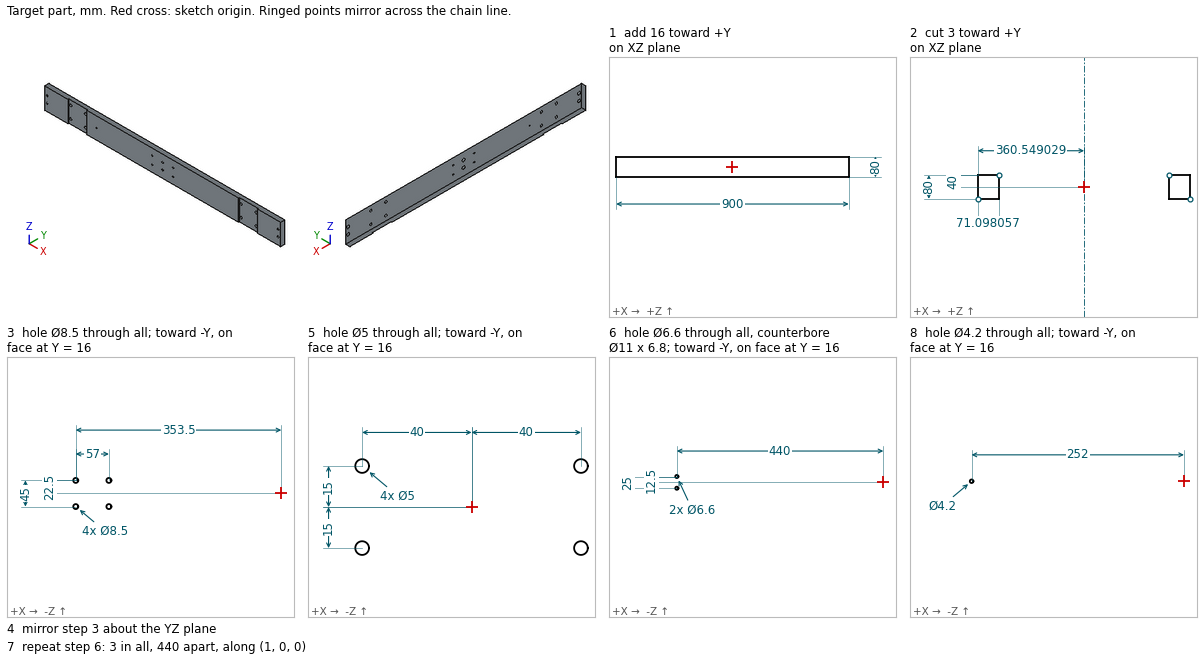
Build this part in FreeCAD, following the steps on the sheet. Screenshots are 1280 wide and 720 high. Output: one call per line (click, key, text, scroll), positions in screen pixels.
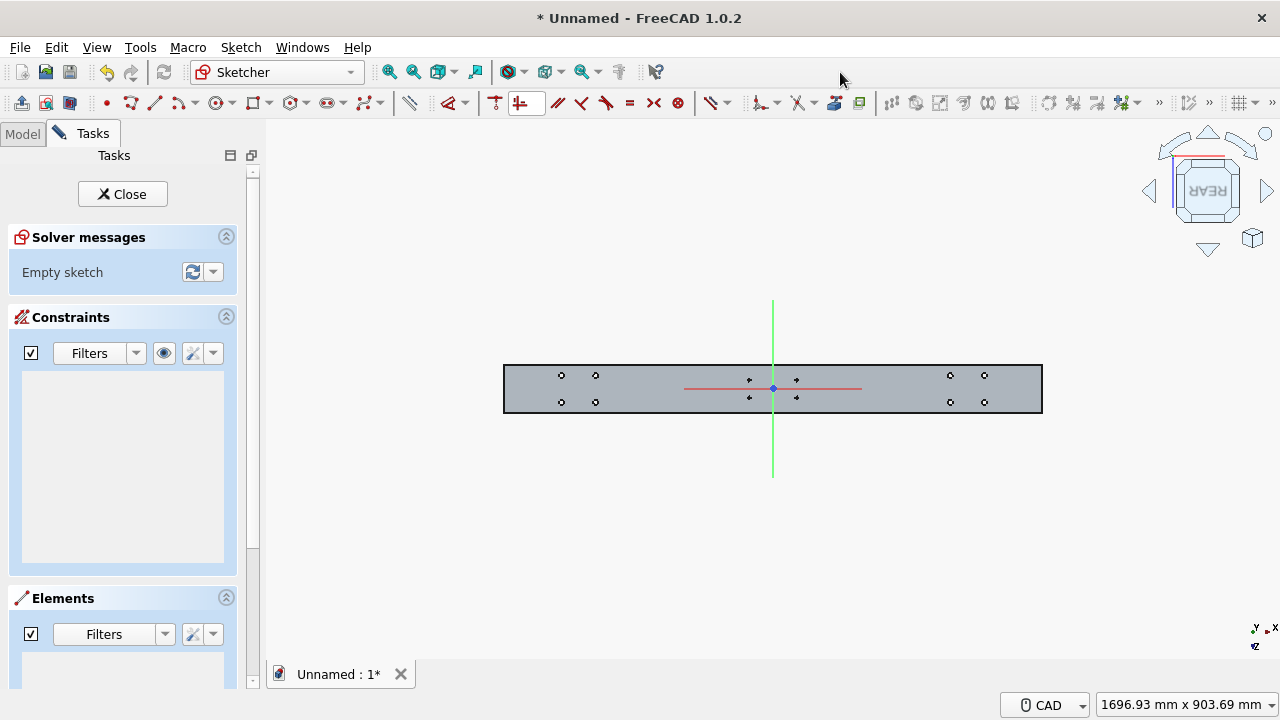
scroll(497, 389, up, 14)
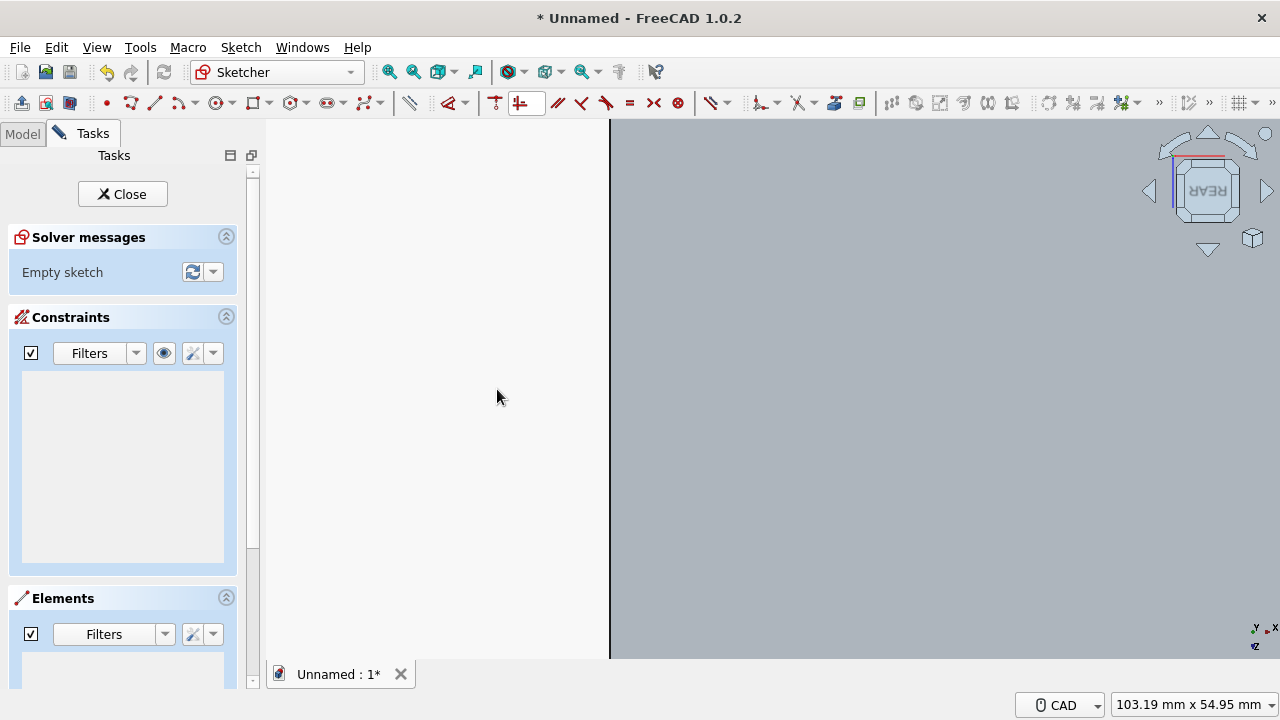
key(g)
key(c)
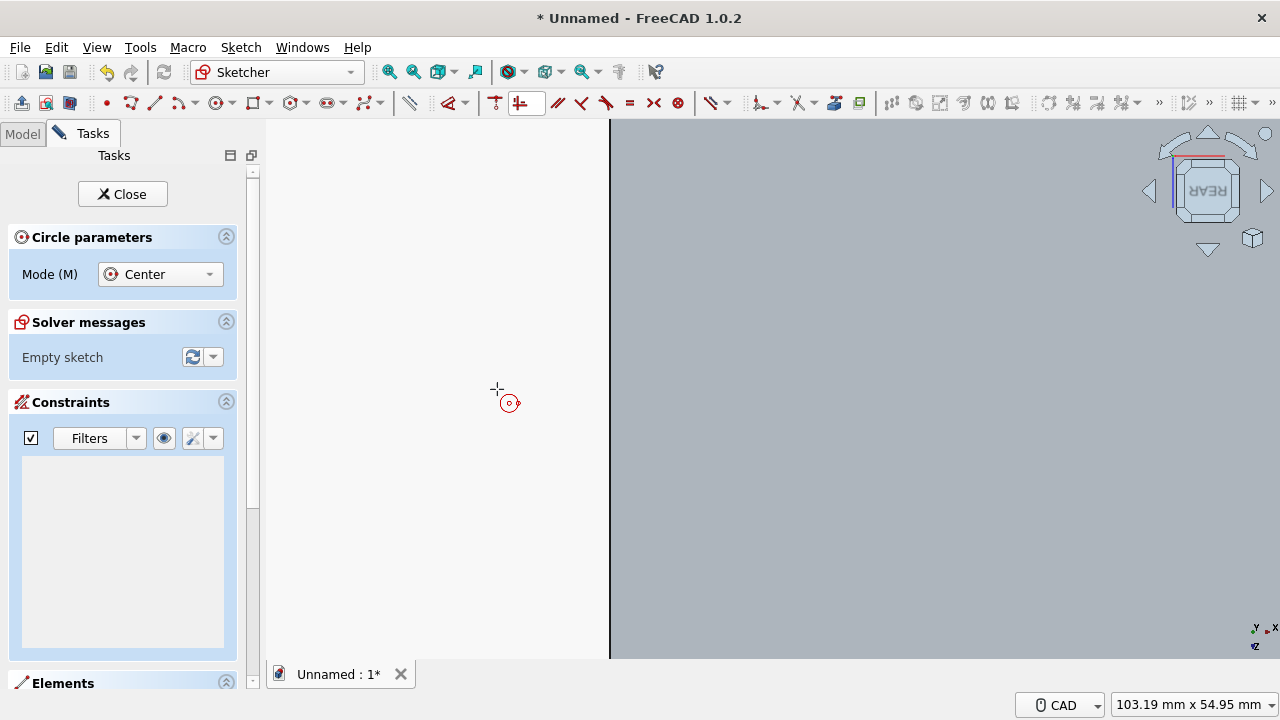
click(709, 258)
click(731, 236)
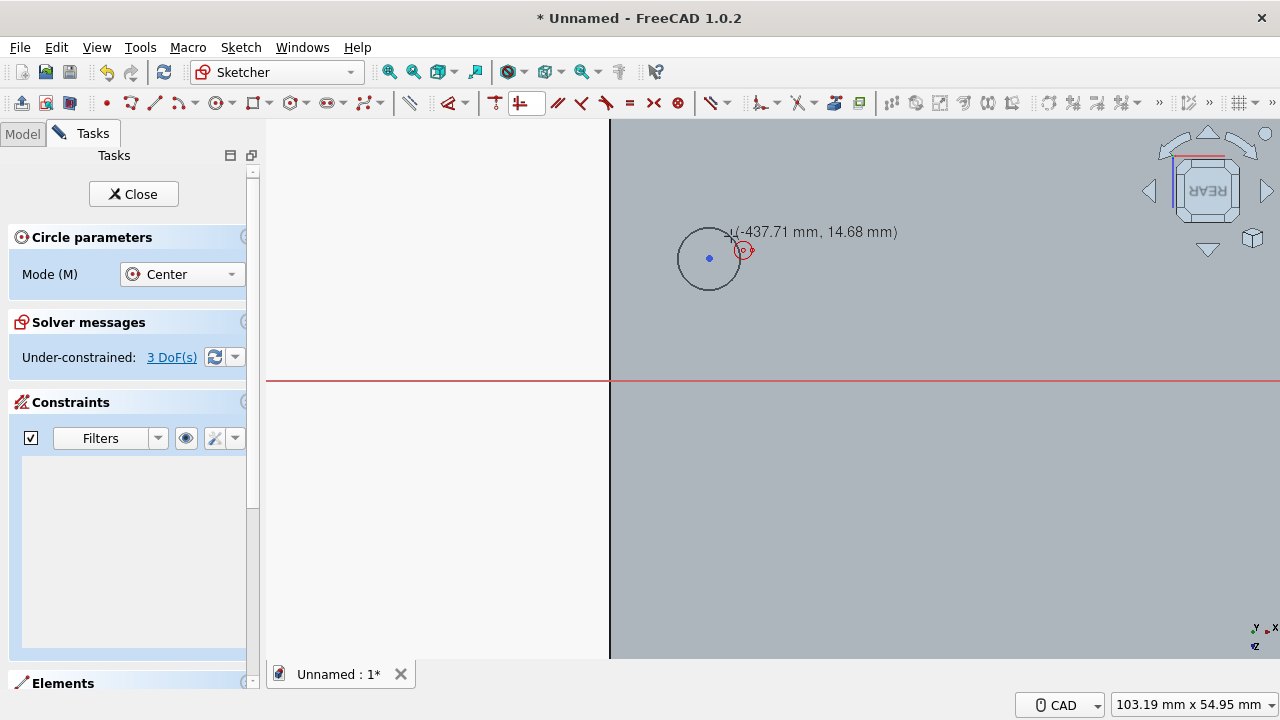
click(709, 504)
click(731, 481)
key(Escape)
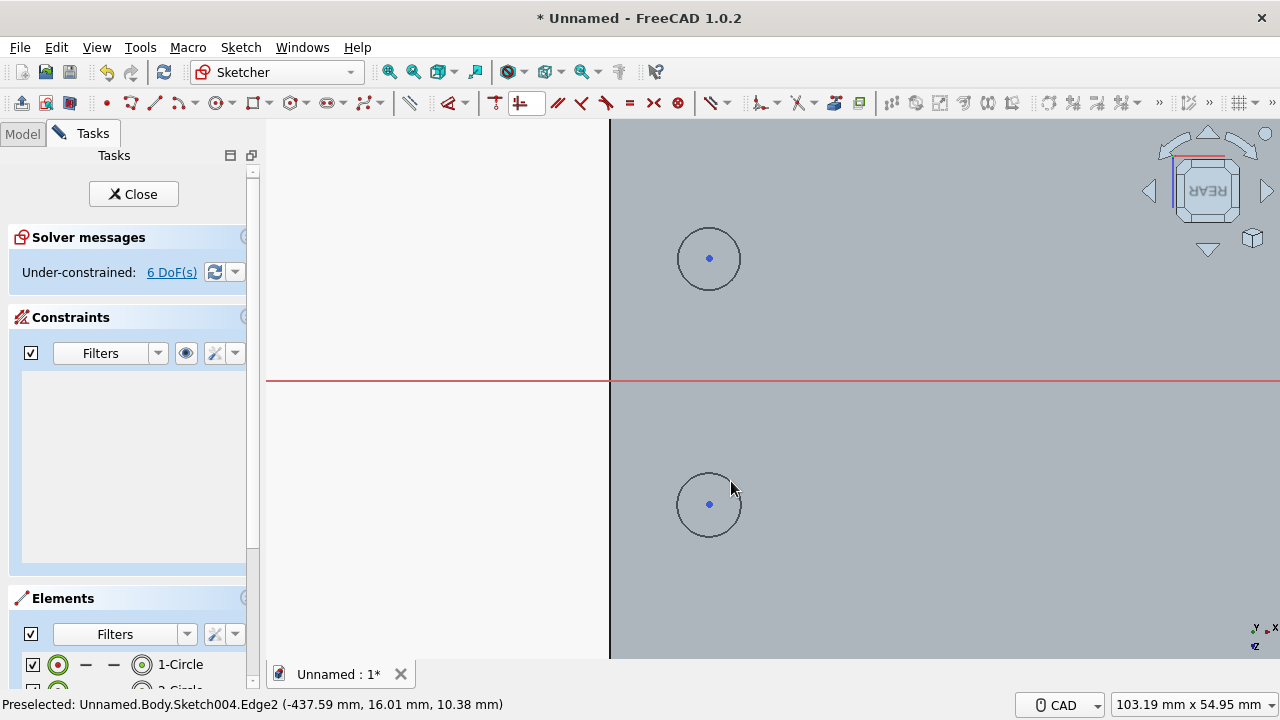
click(731, 237)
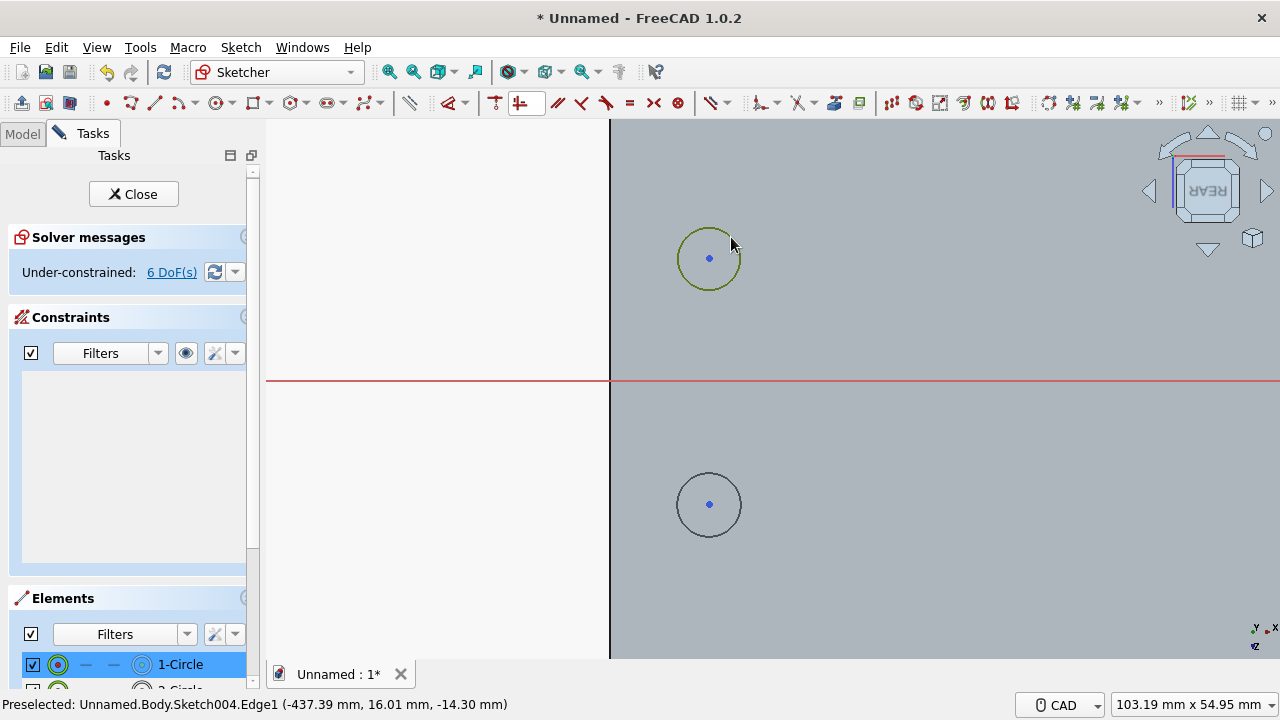
click(731, 482)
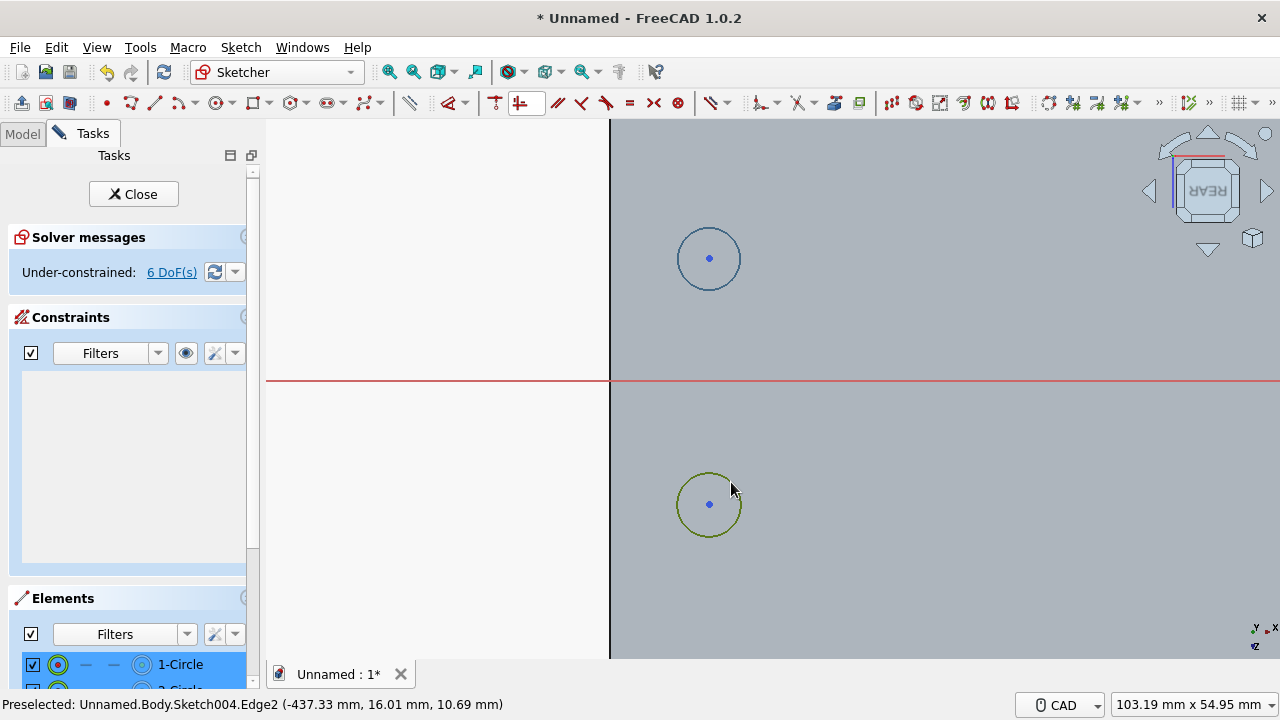
key(e)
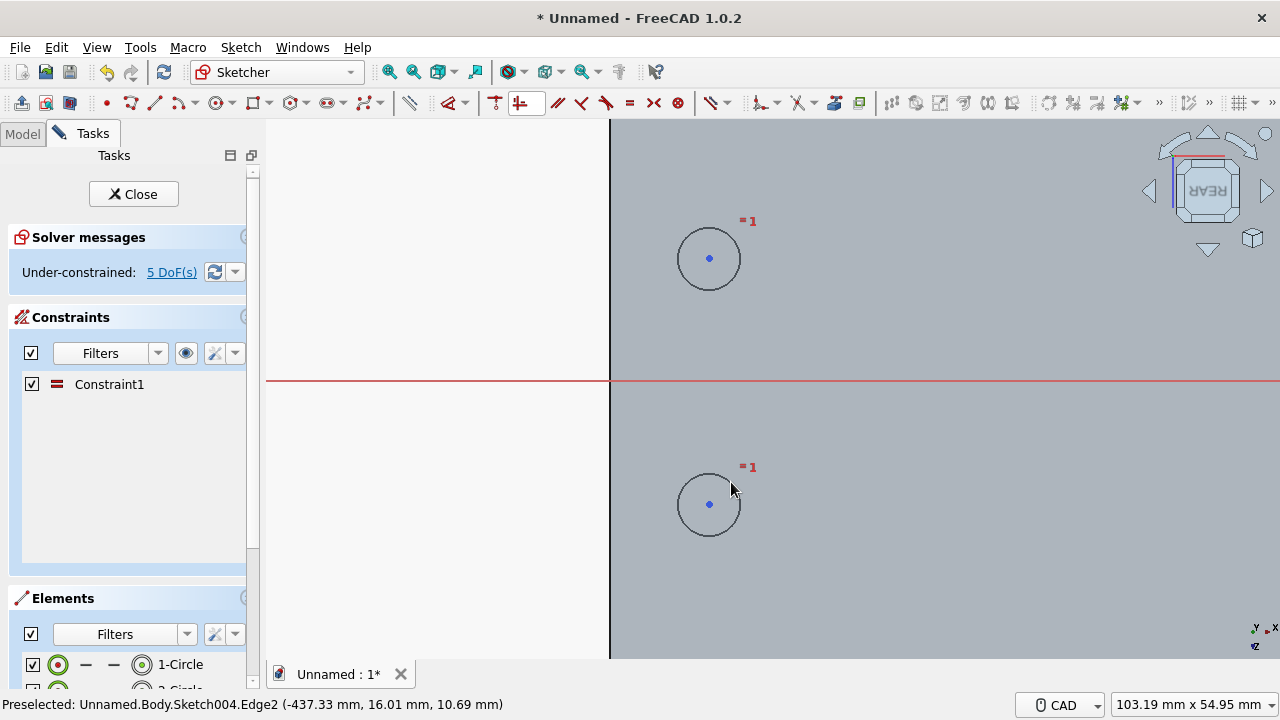
click(709, 259)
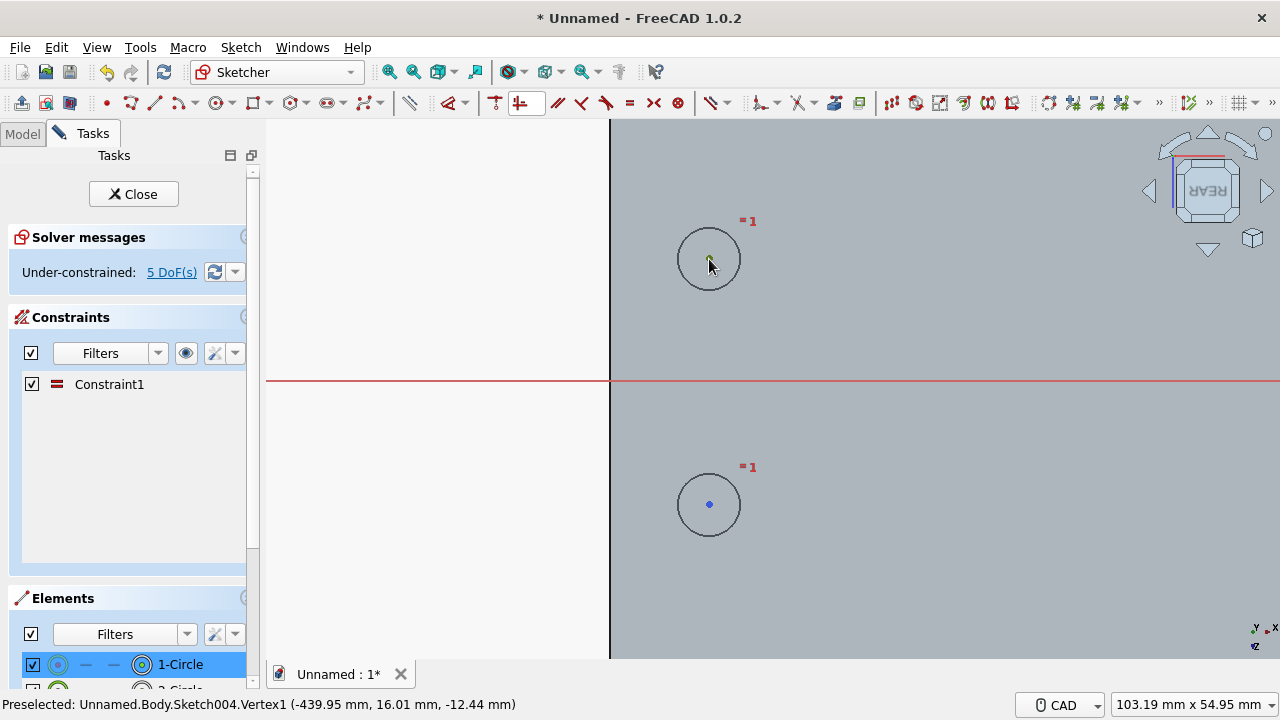
click(709, 505)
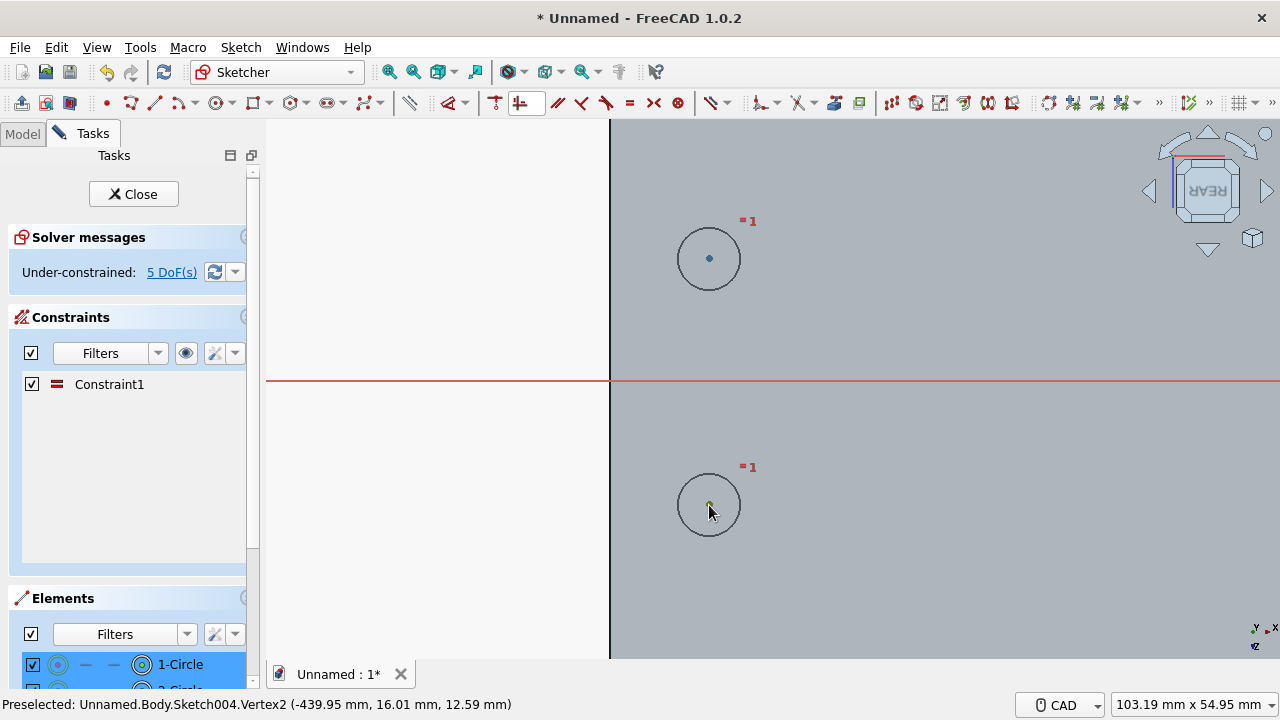
key(v)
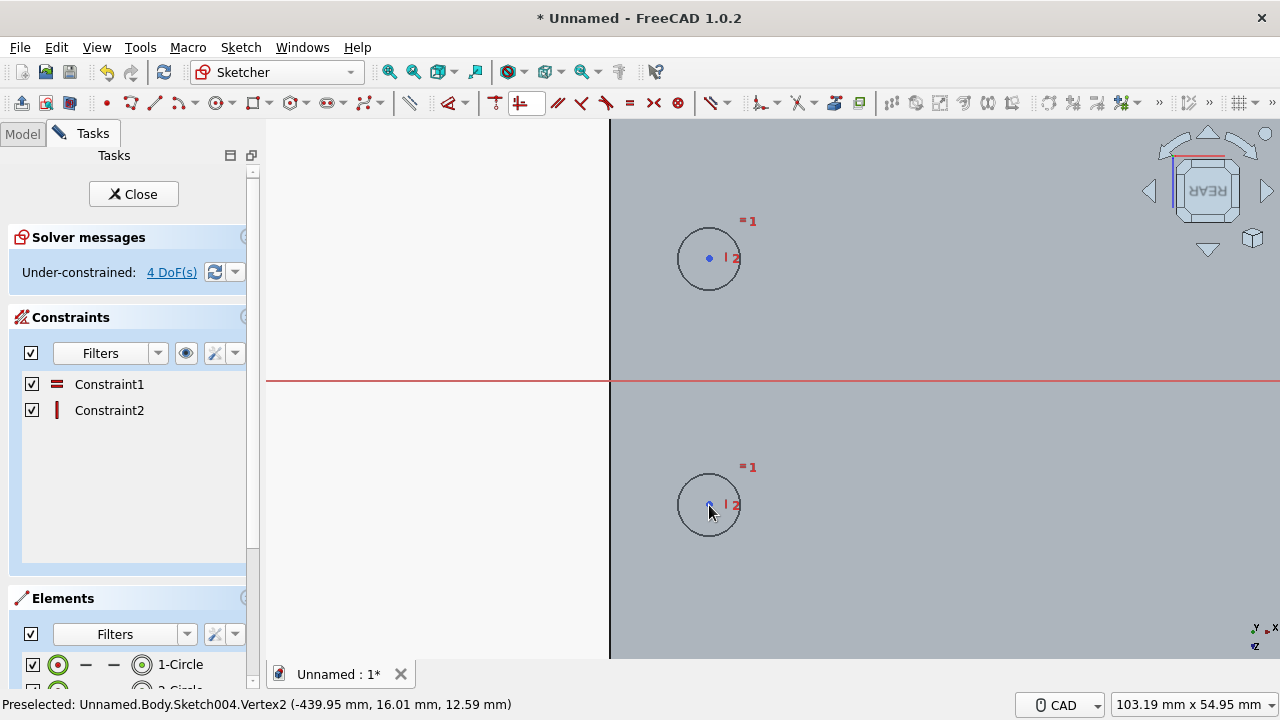
click(448, 104)